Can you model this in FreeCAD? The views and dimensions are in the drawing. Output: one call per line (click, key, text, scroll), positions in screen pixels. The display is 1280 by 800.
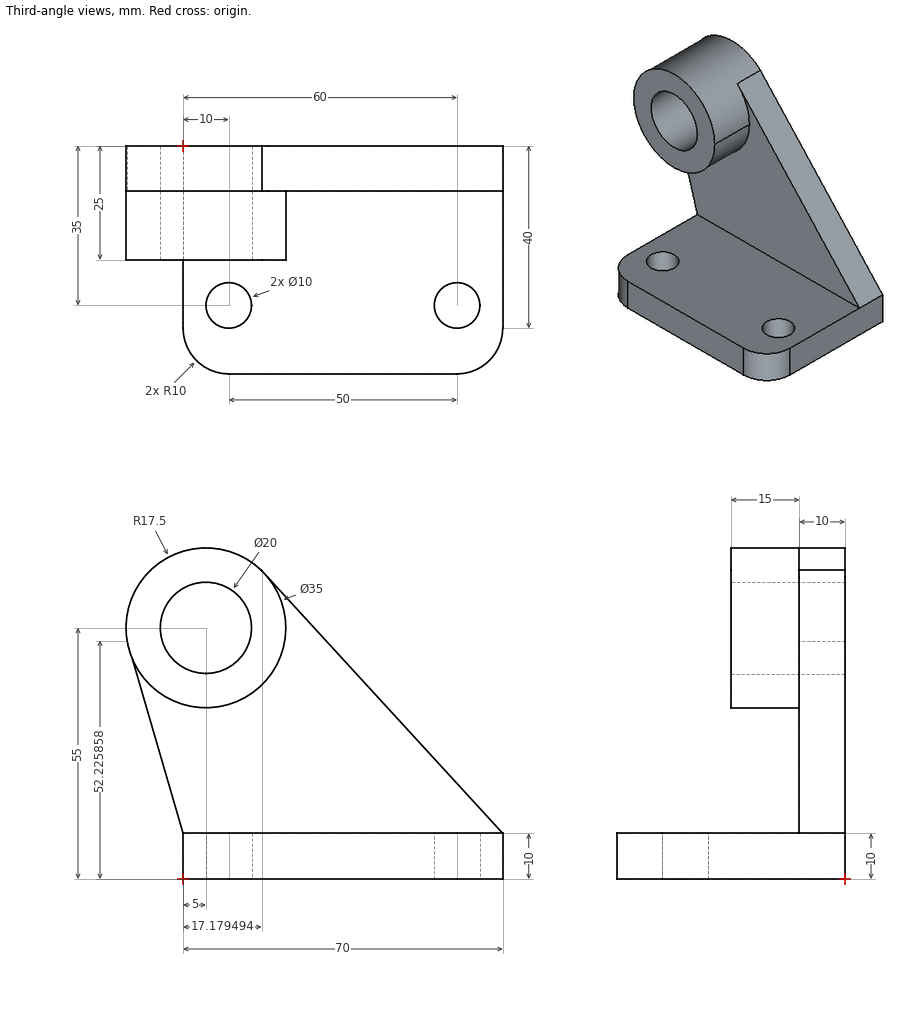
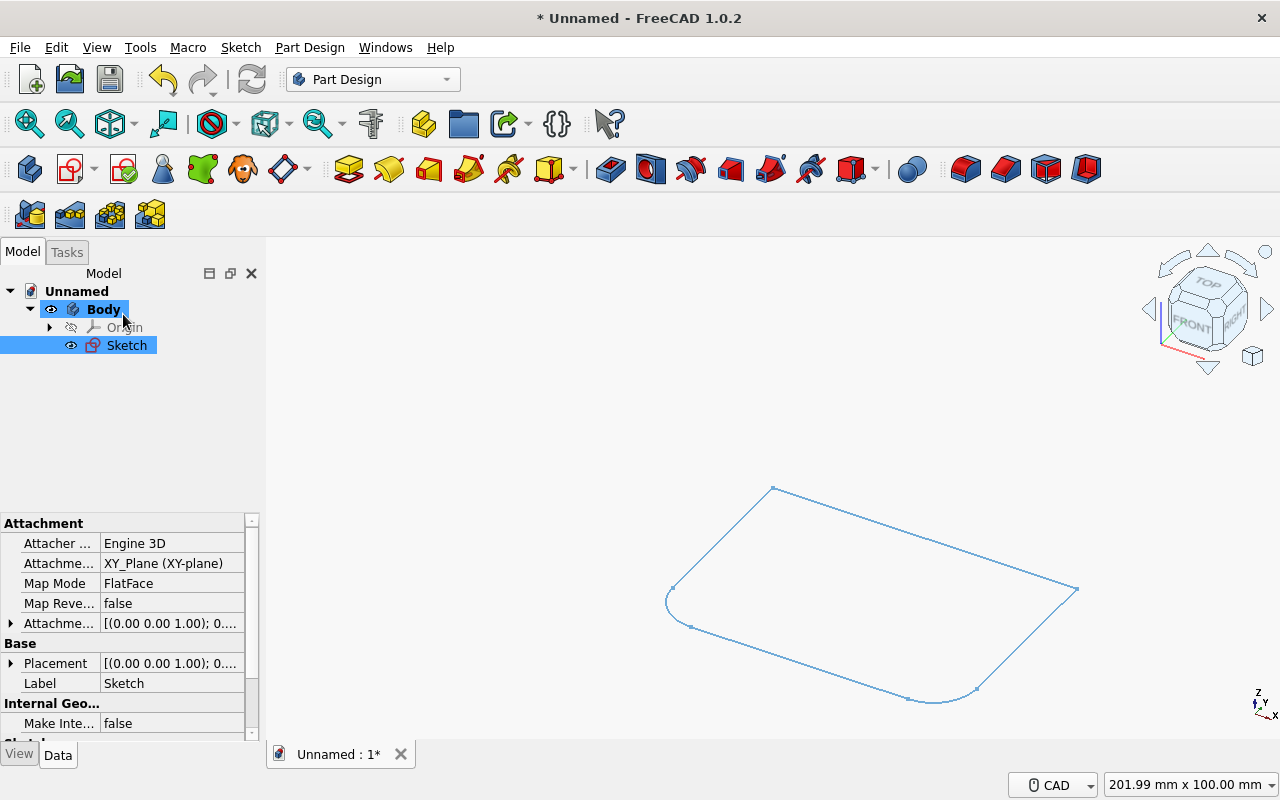
click(350, 170)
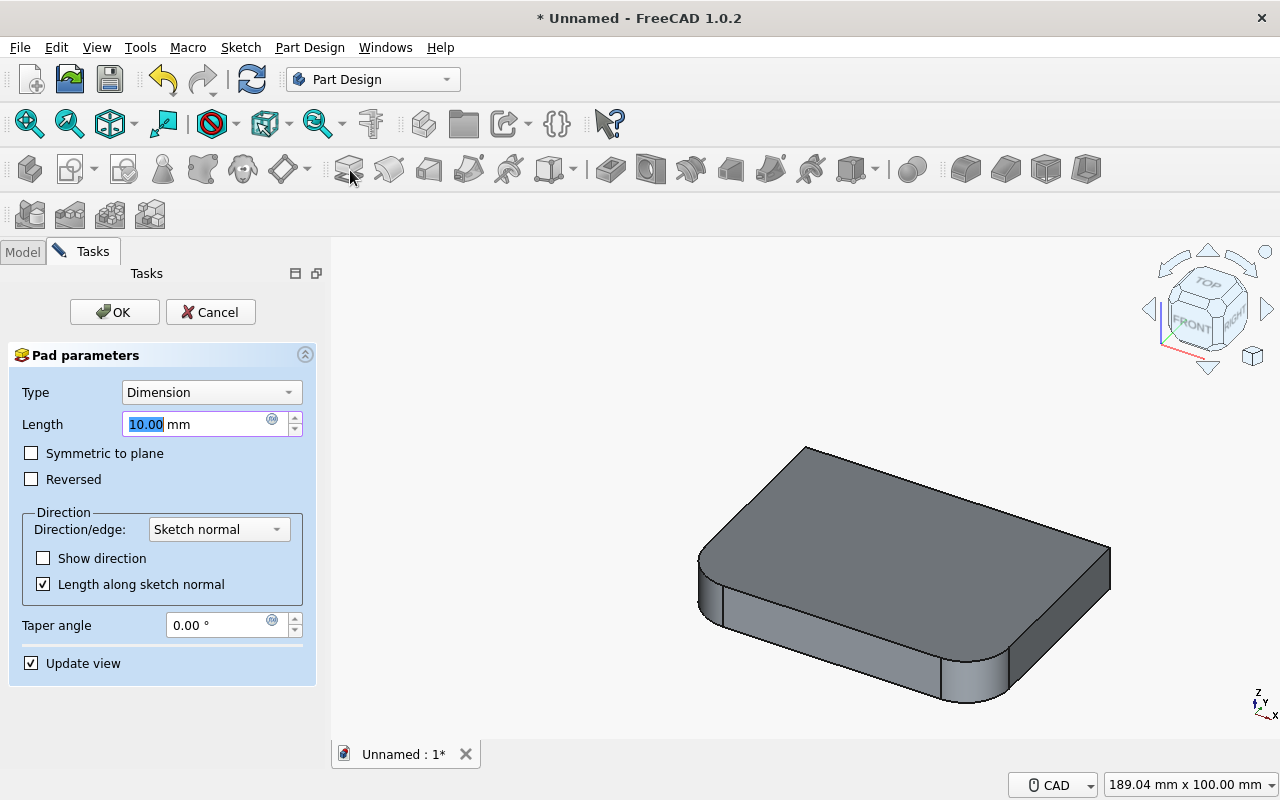
text(10)
key(Tab)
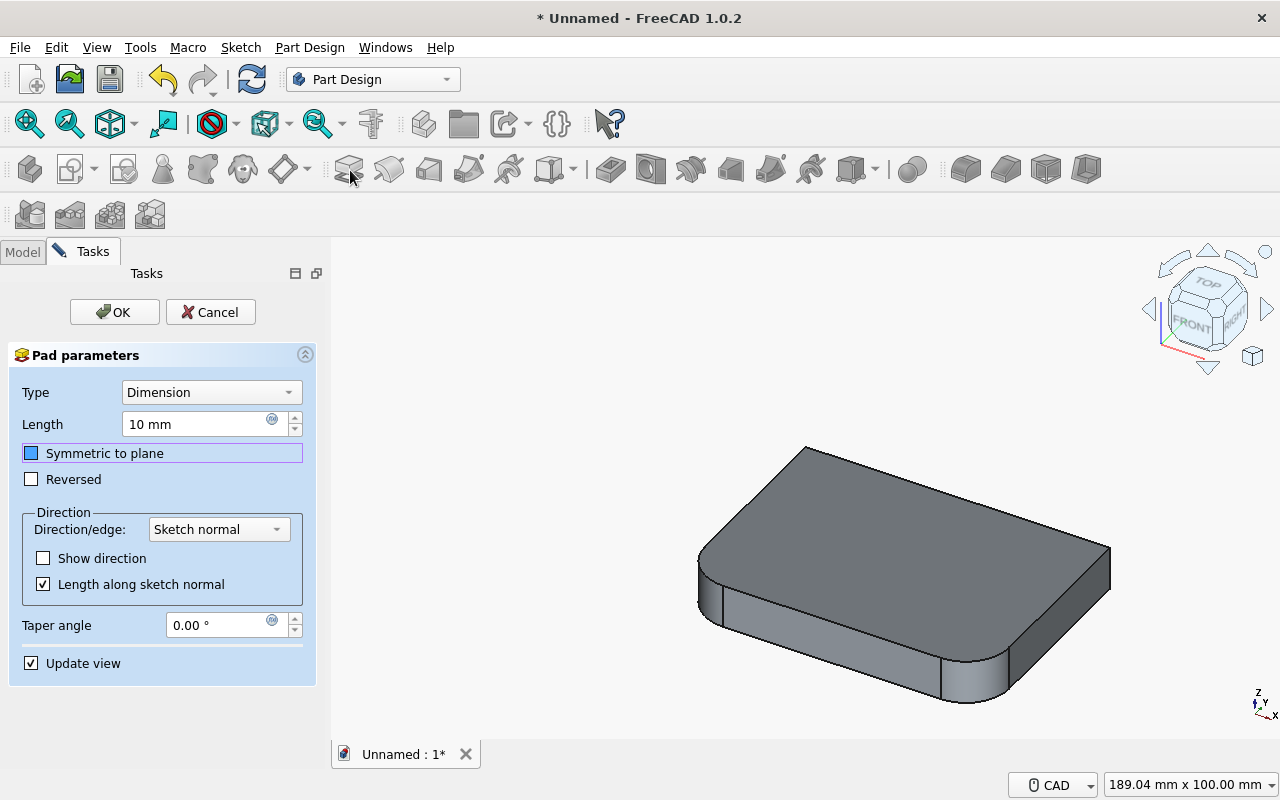
click(115, 312)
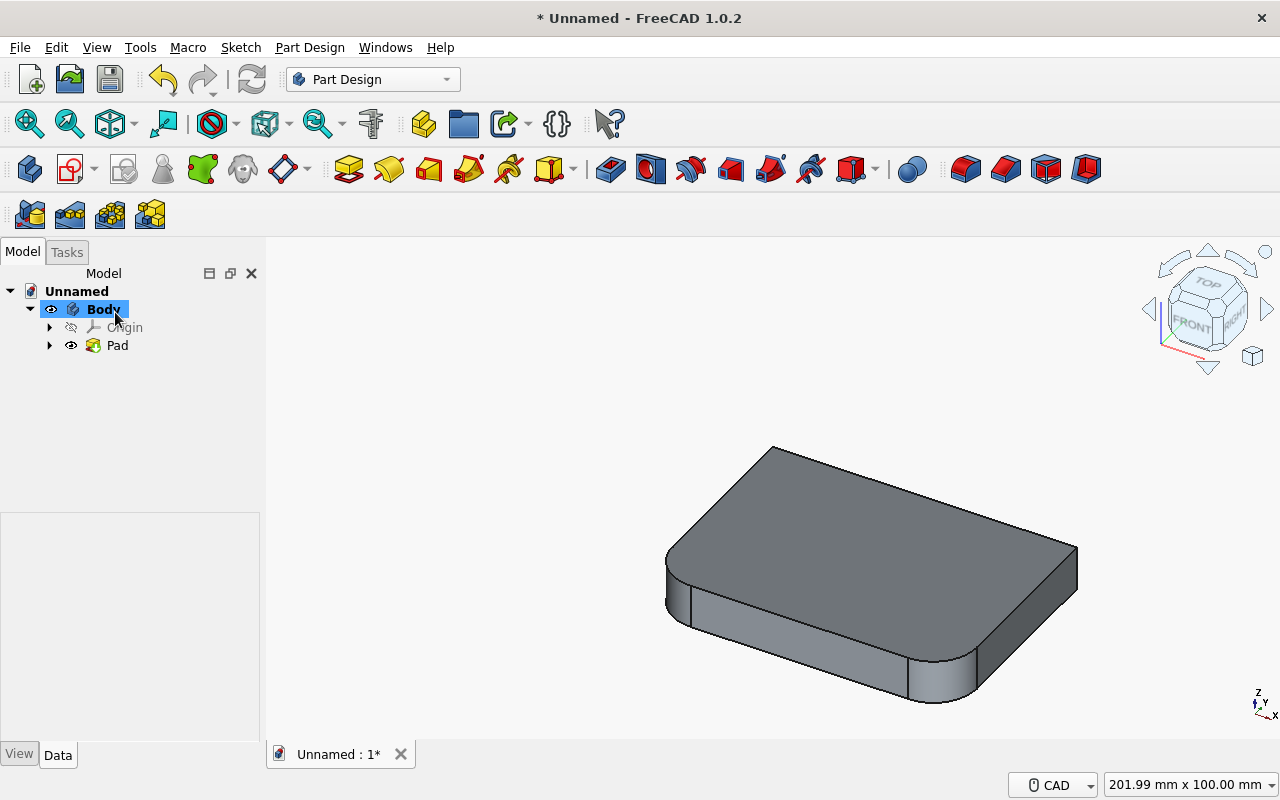
click(70, 170)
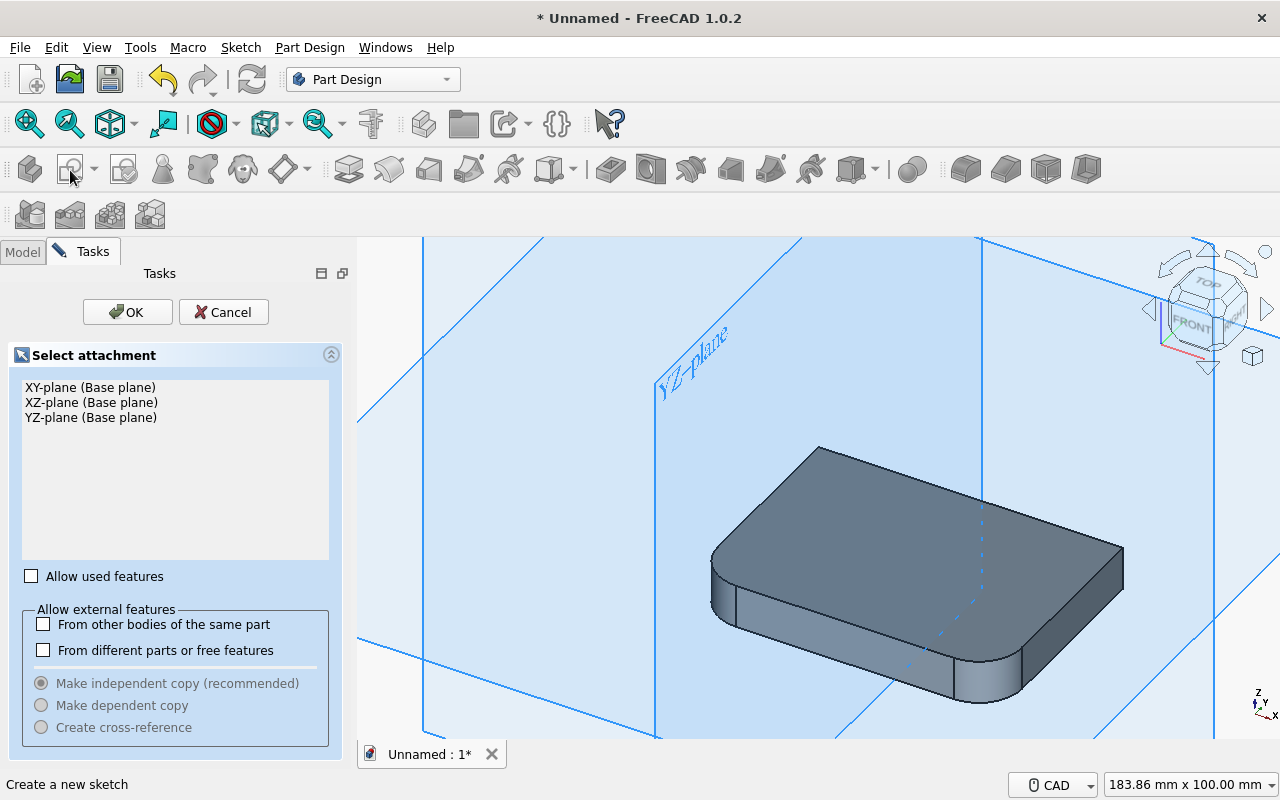
click(82, 402)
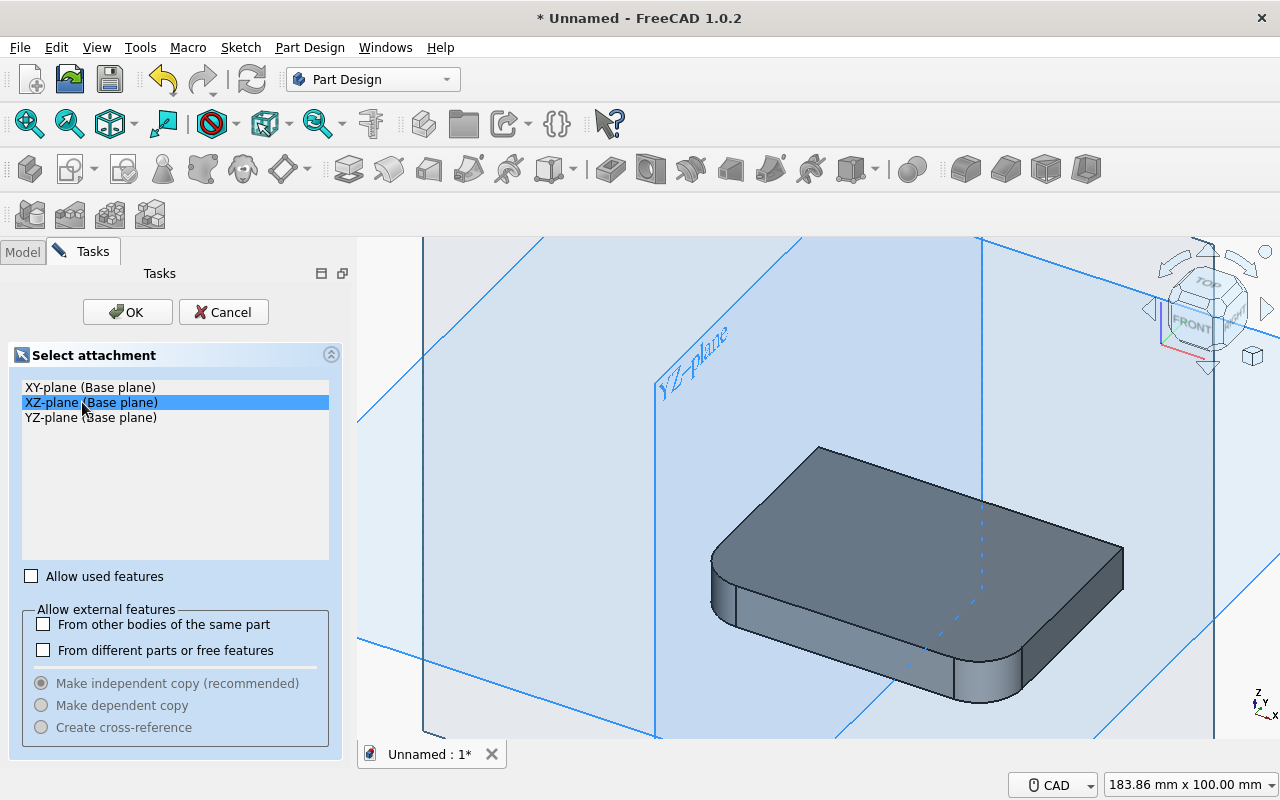
click(128, 312)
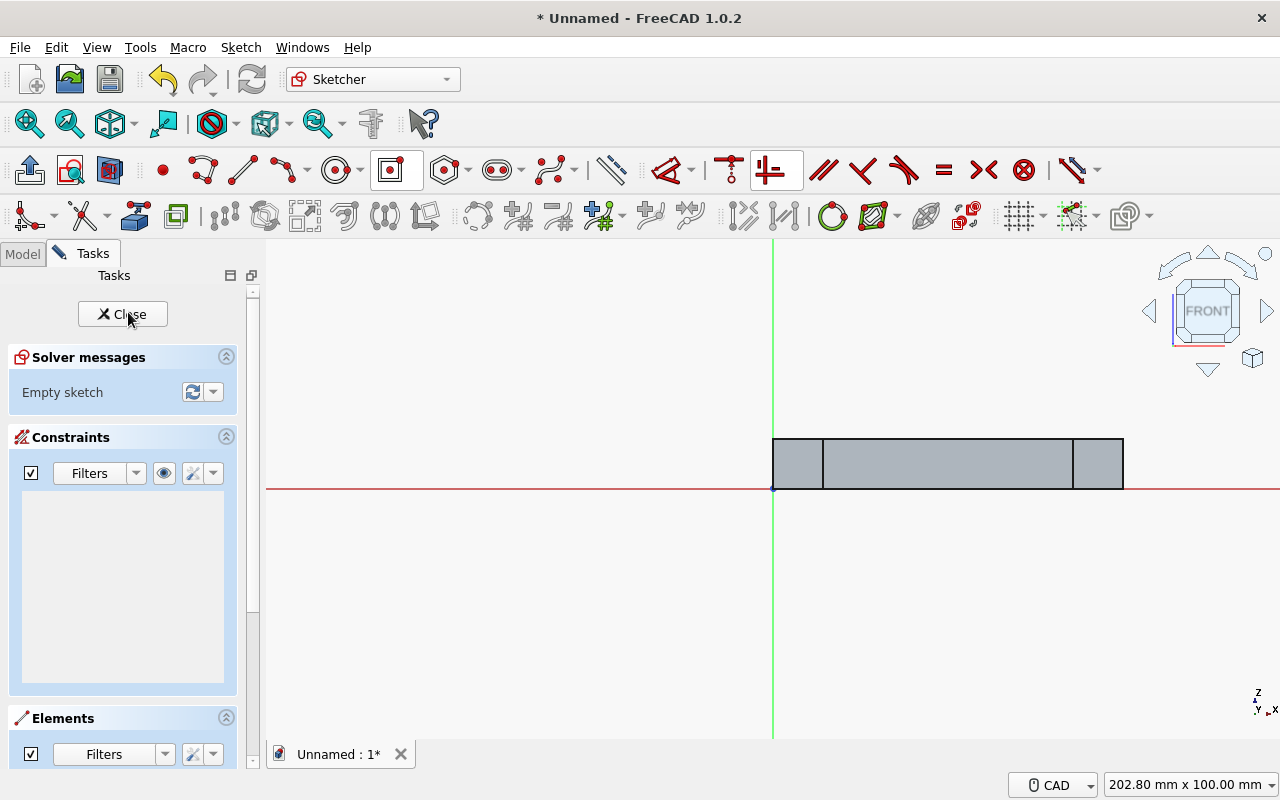
click(110, 170)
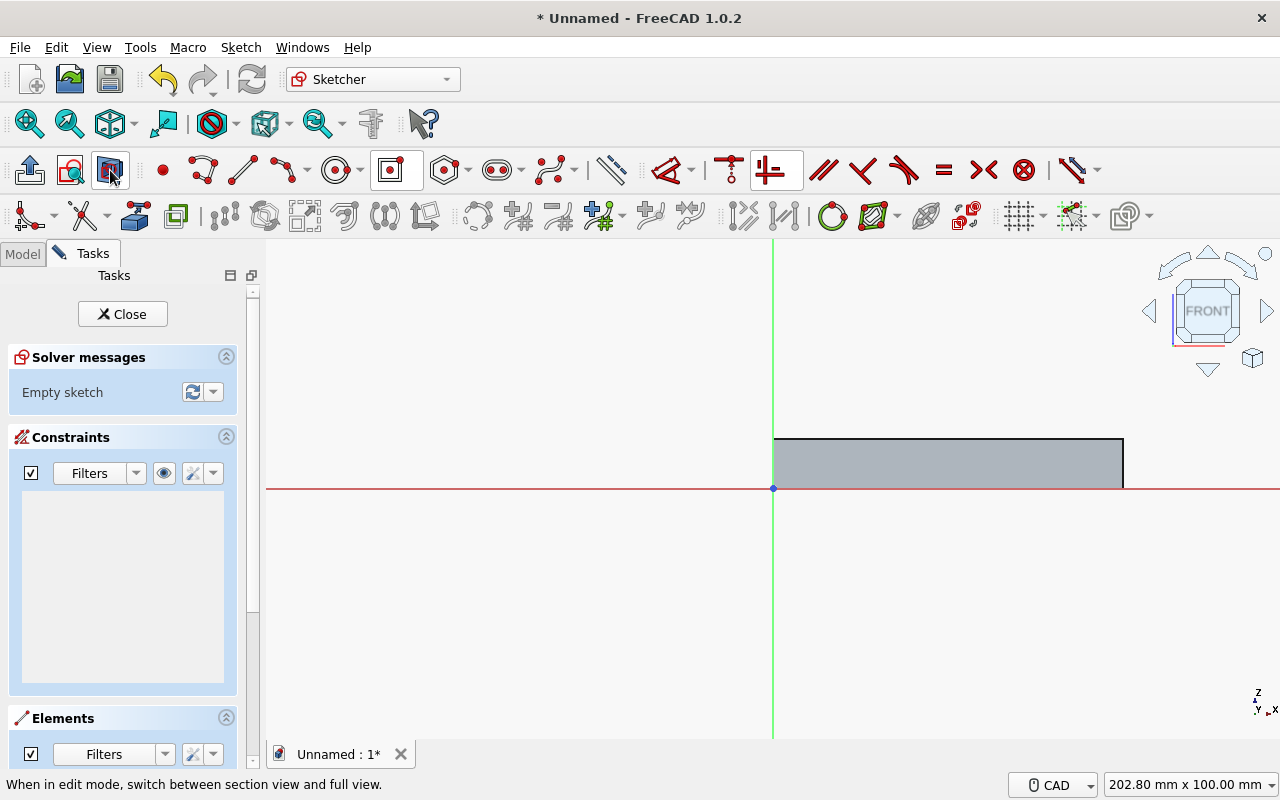
scroll(294, 711, down, 2)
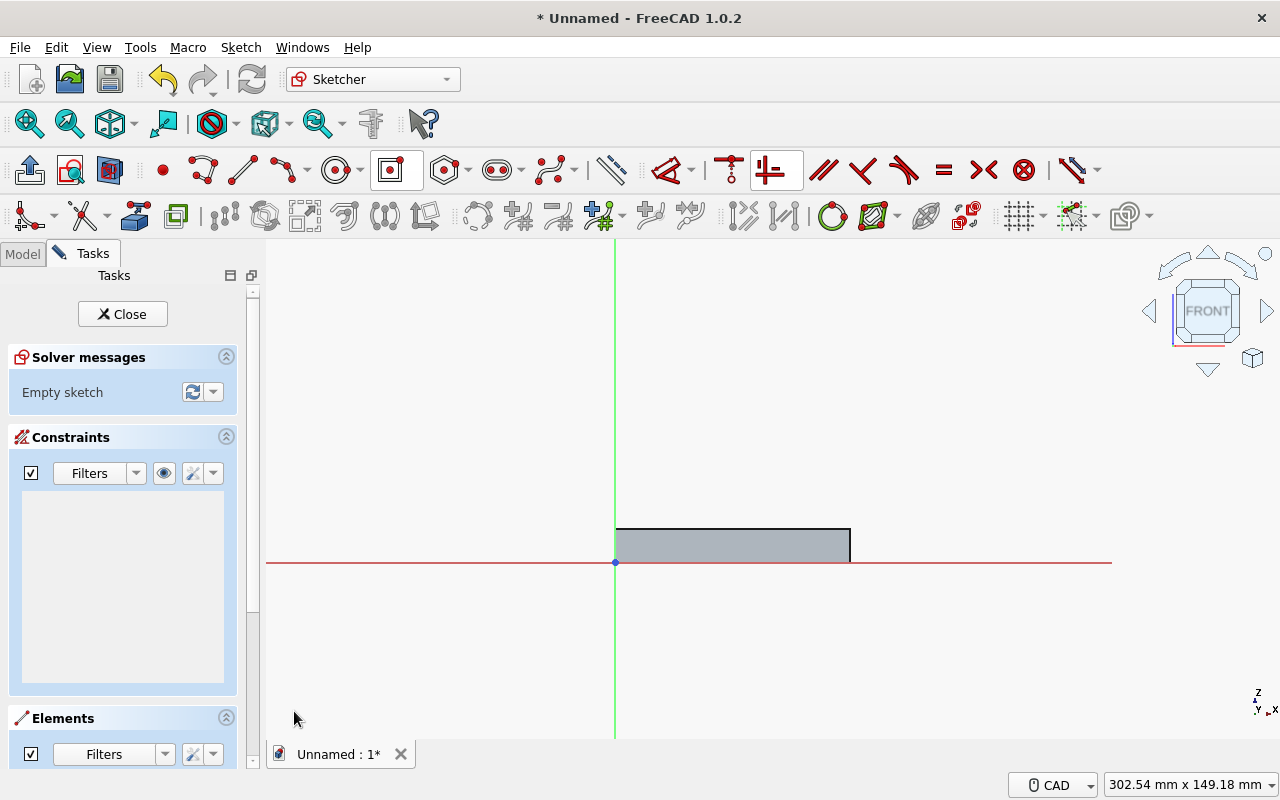
click(204, 170)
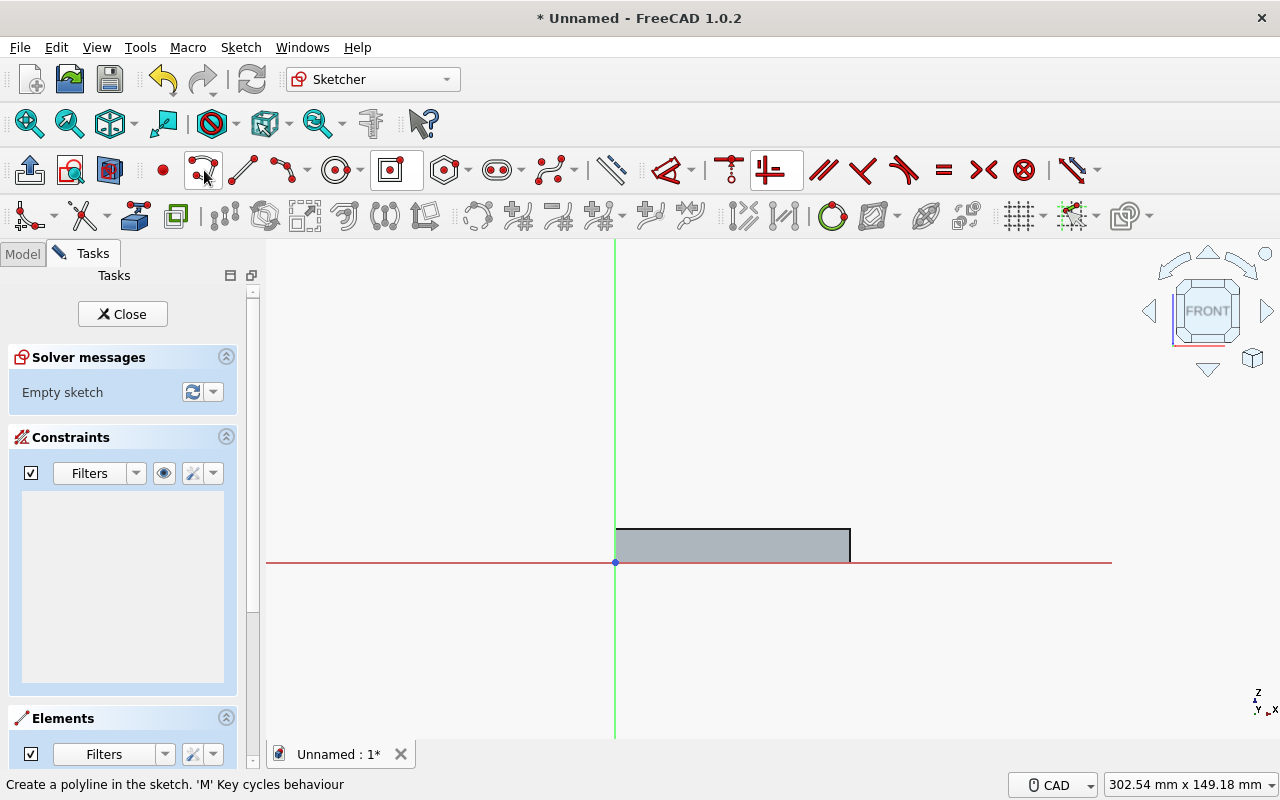
click(673, 336)
click(850, 529)
click(615, 529)
click(574, 387)
right_click(574, 387)